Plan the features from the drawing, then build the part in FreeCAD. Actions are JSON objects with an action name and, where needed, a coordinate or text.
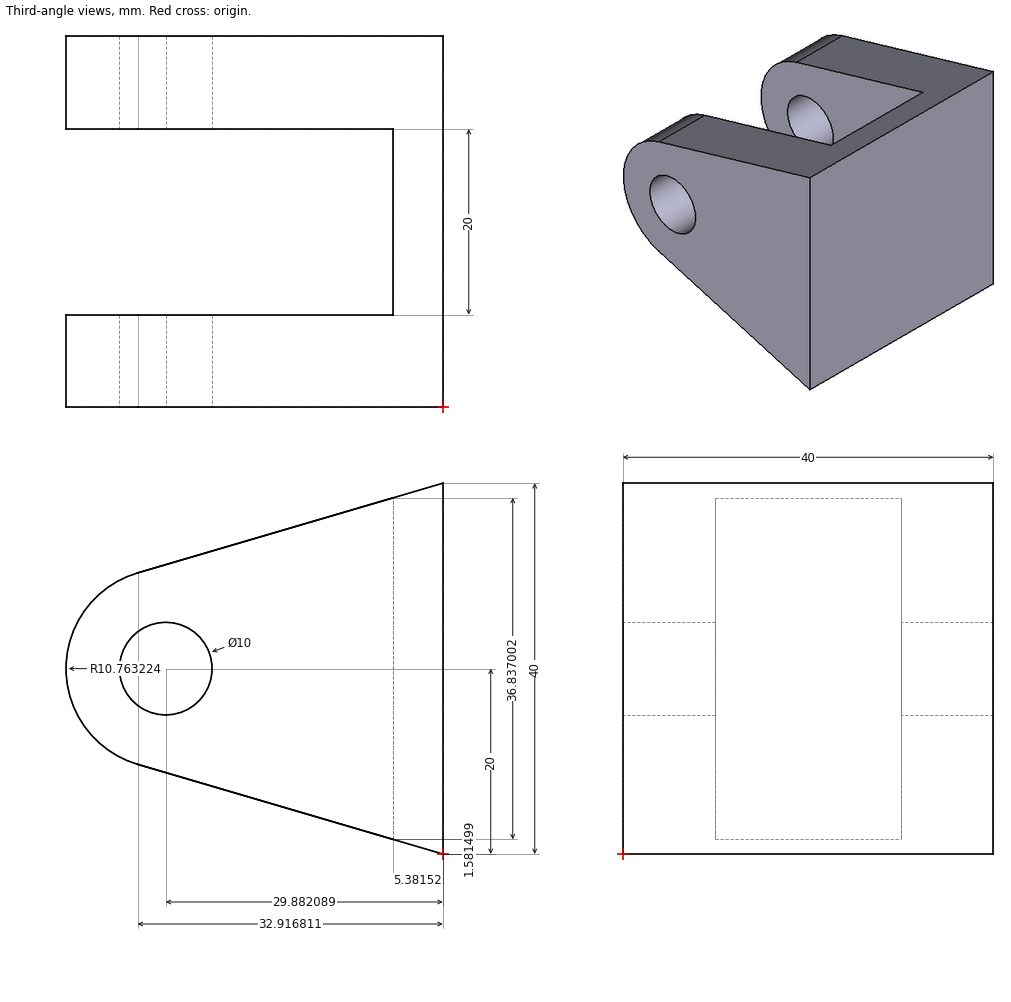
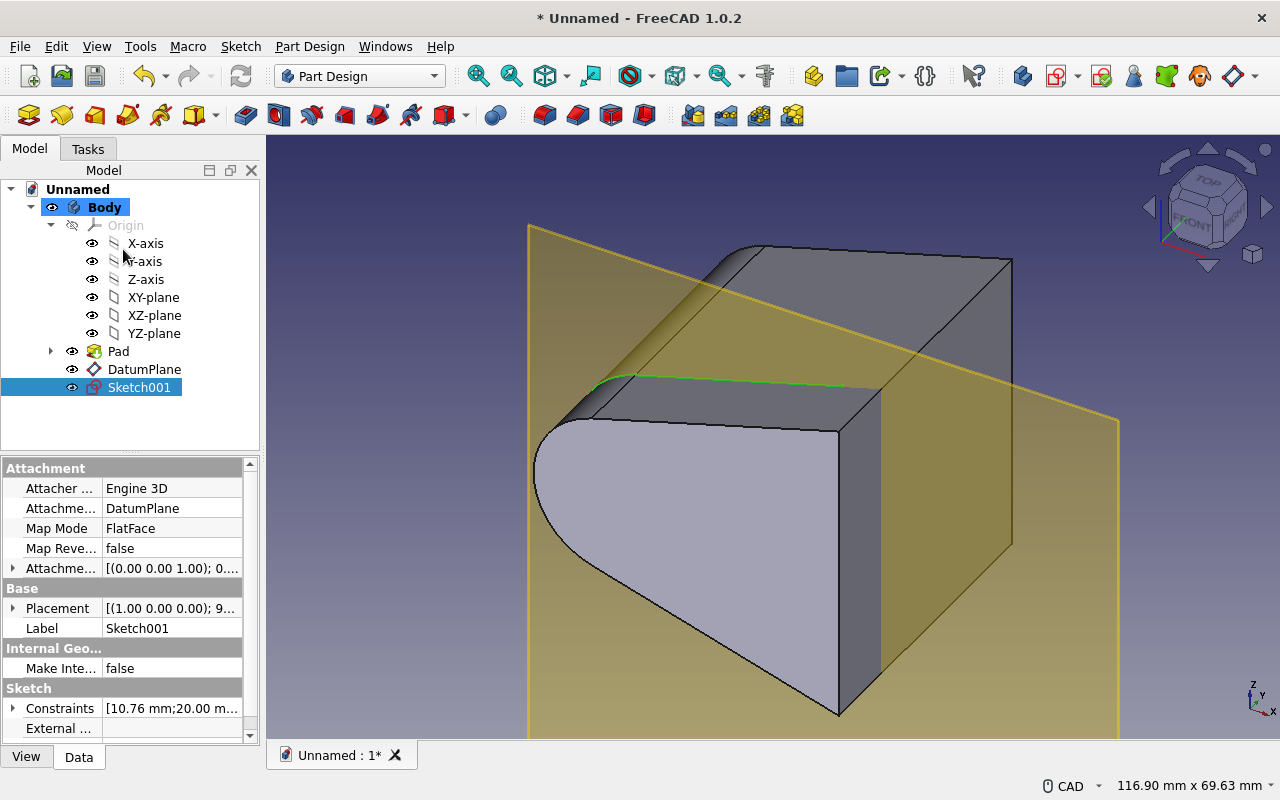
{"action": "left_click", "coordinate": [246, 116]}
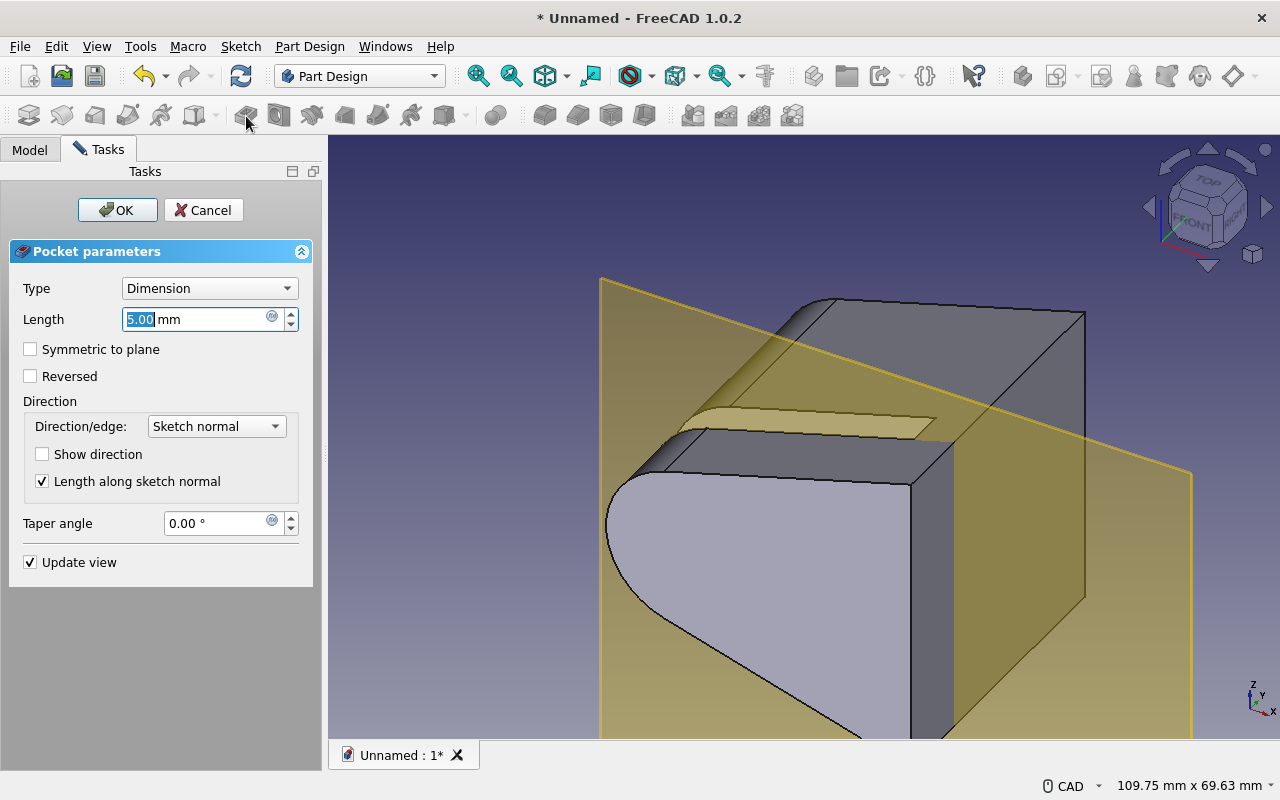
{"action": "type", "text": "20"}
{"action": "key", "text": "Tab"}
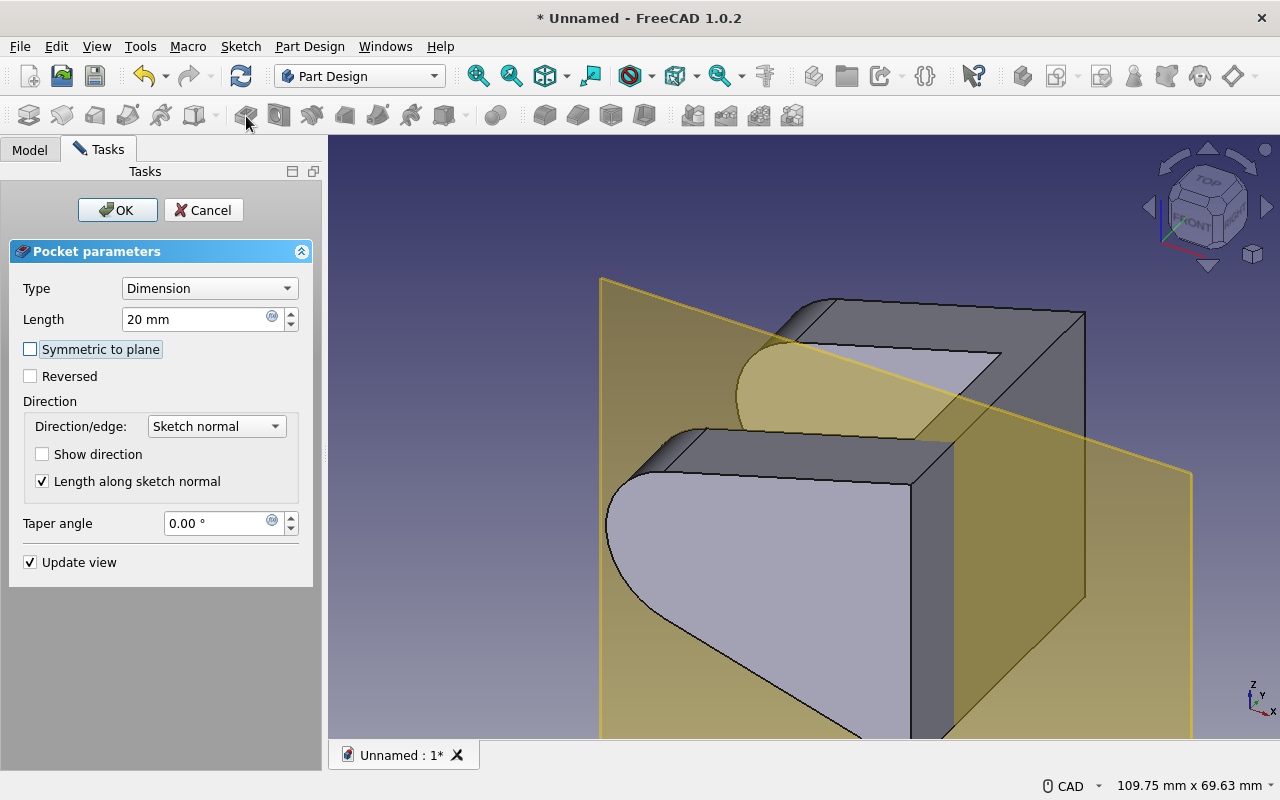
{"action": "left_click", "coordinate": [118, 210]}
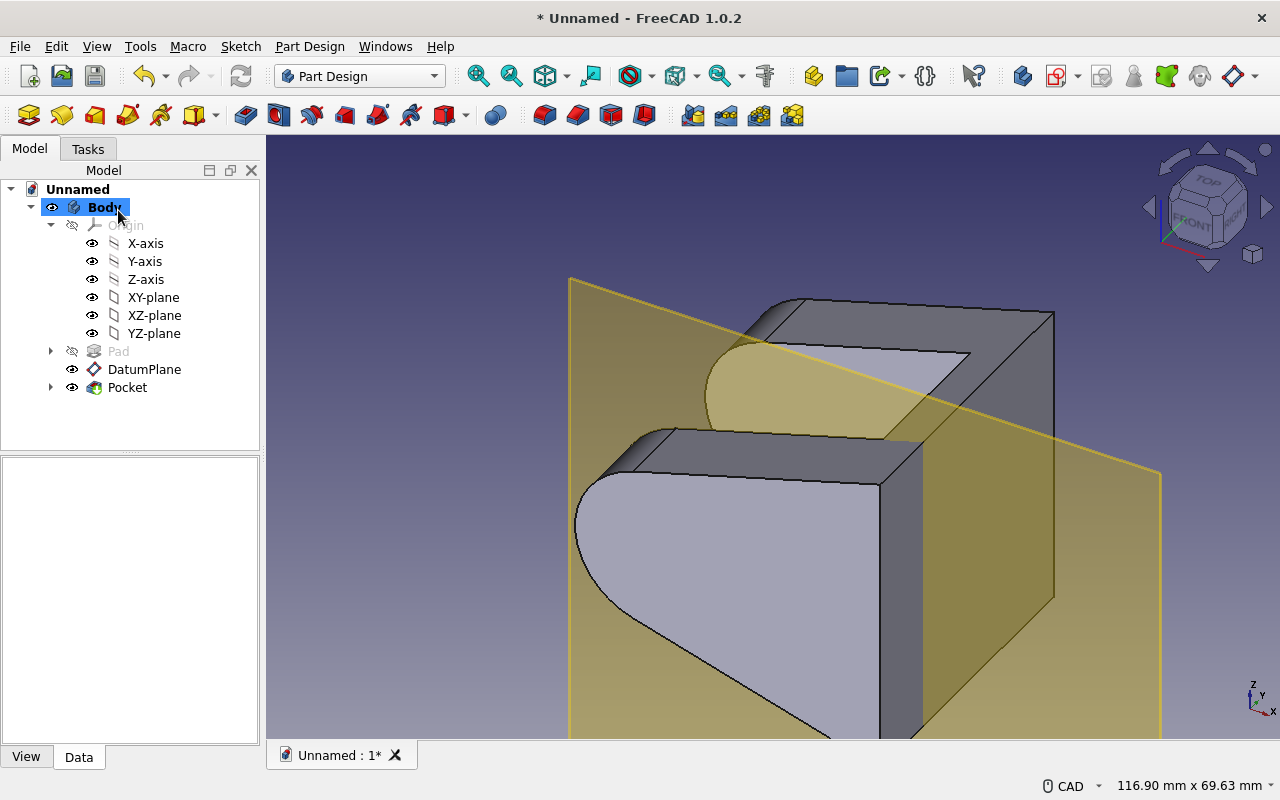
{"action": "left_click", "coordinate": [117, 369]}
{"action": "key", "text": "space"}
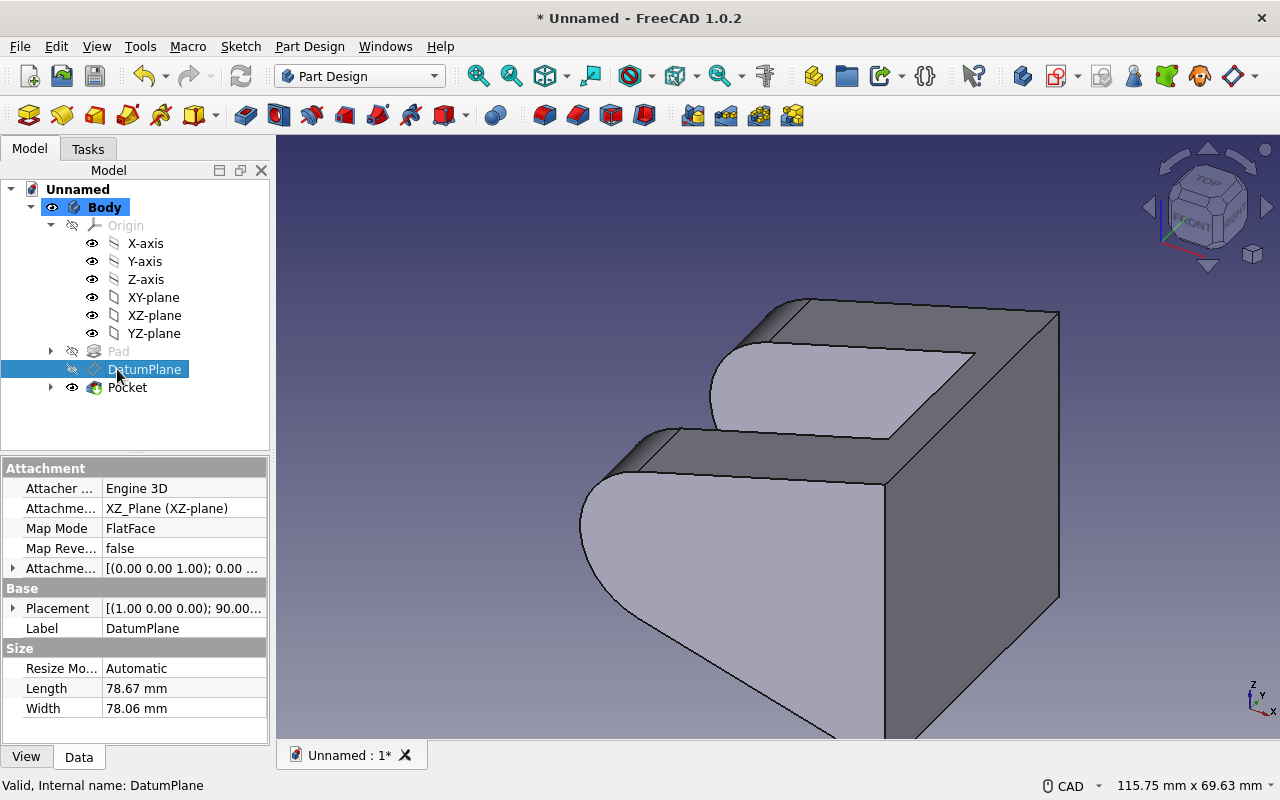
{"action": "left_click", "coordinate": [479, 76]}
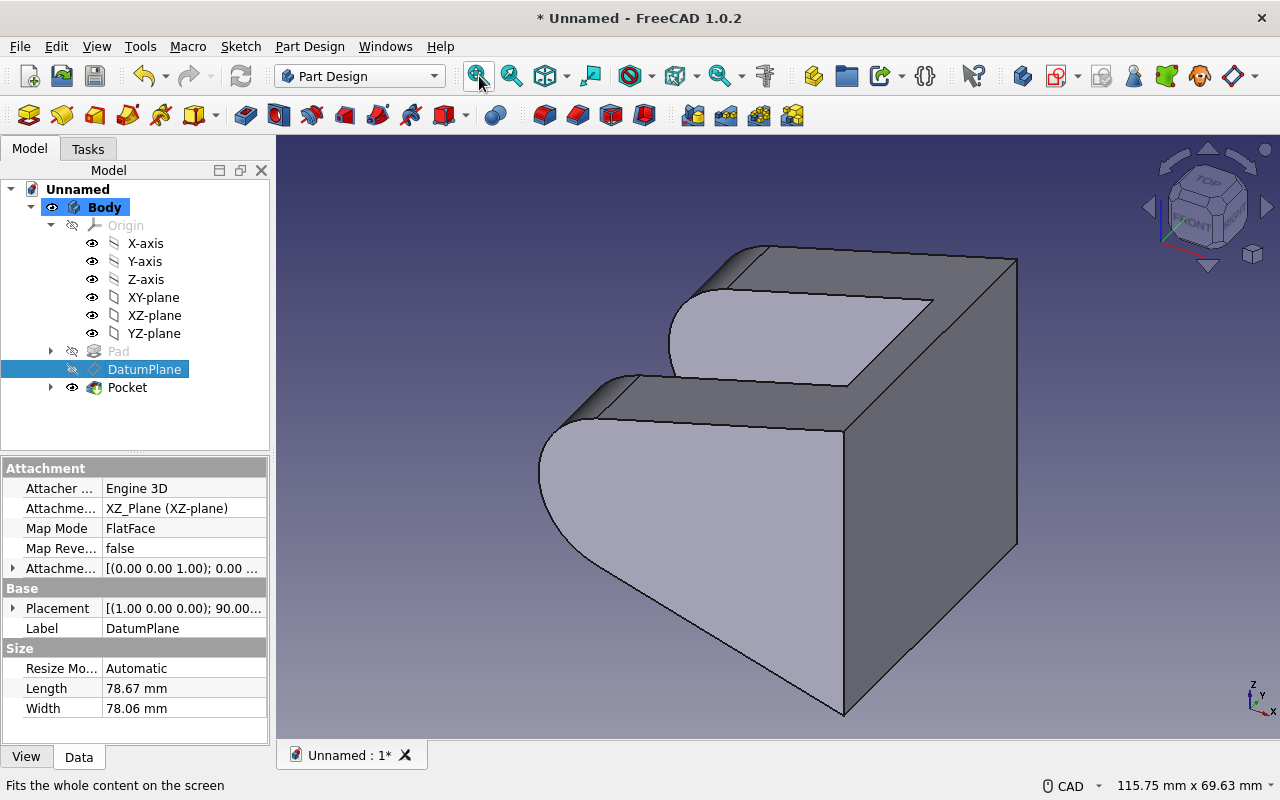
{"action": "left_click", "coordinate": [137, 315]}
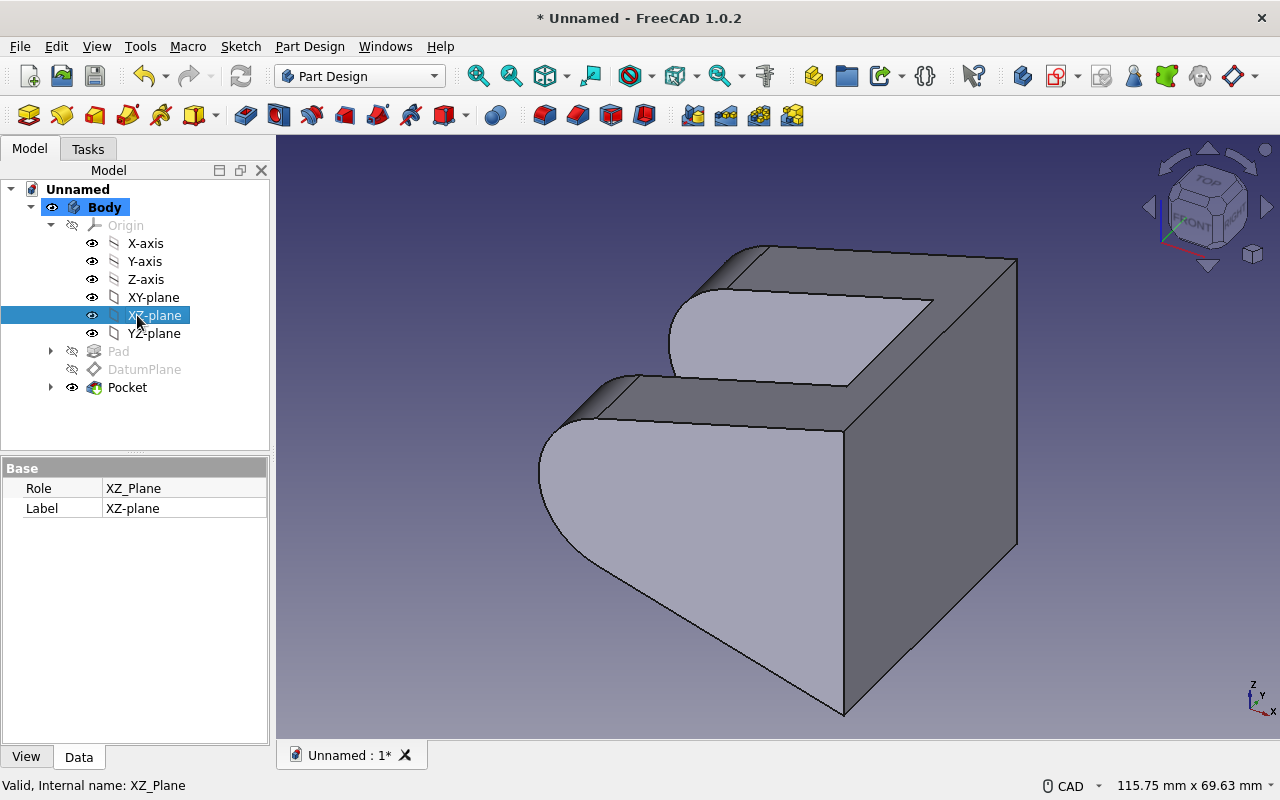
{"action": "left_click", "coordinate": [1232, 76]}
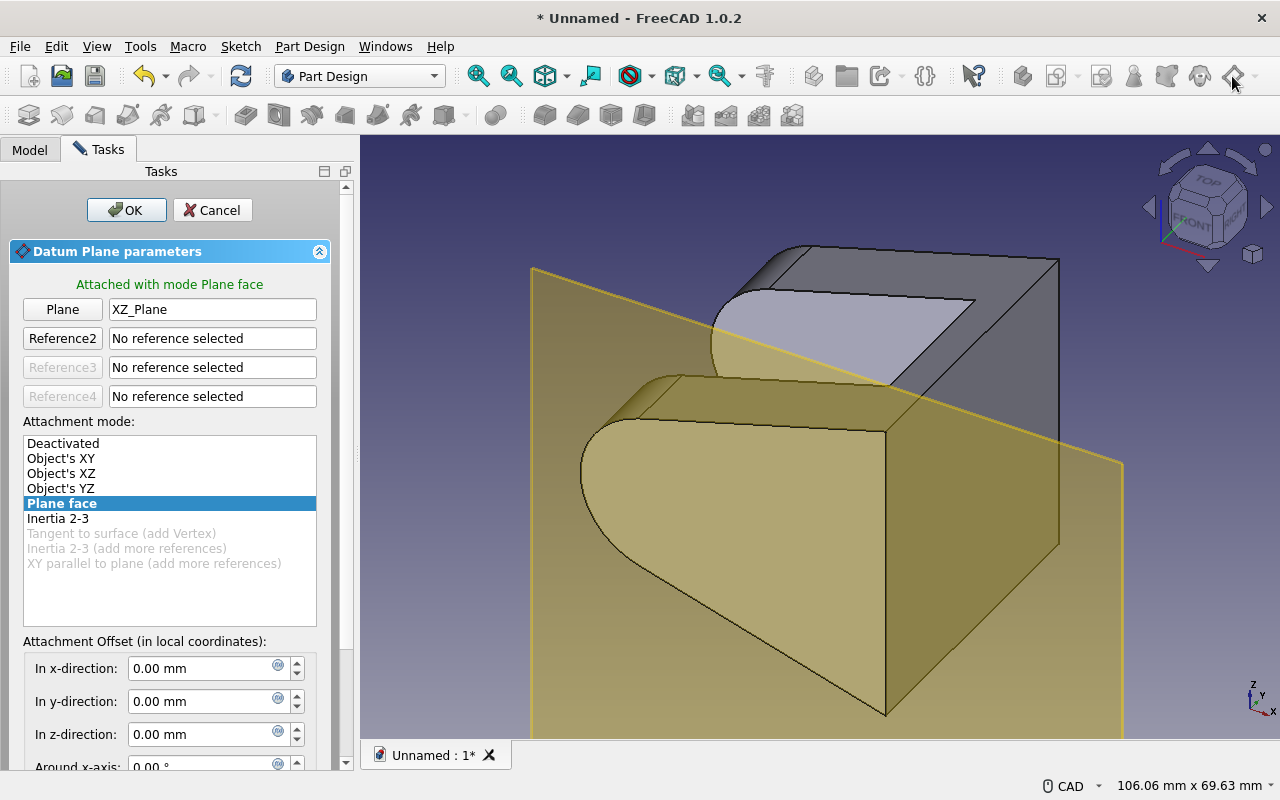
{"action": "triple_click", "coordinate": [210, 734]}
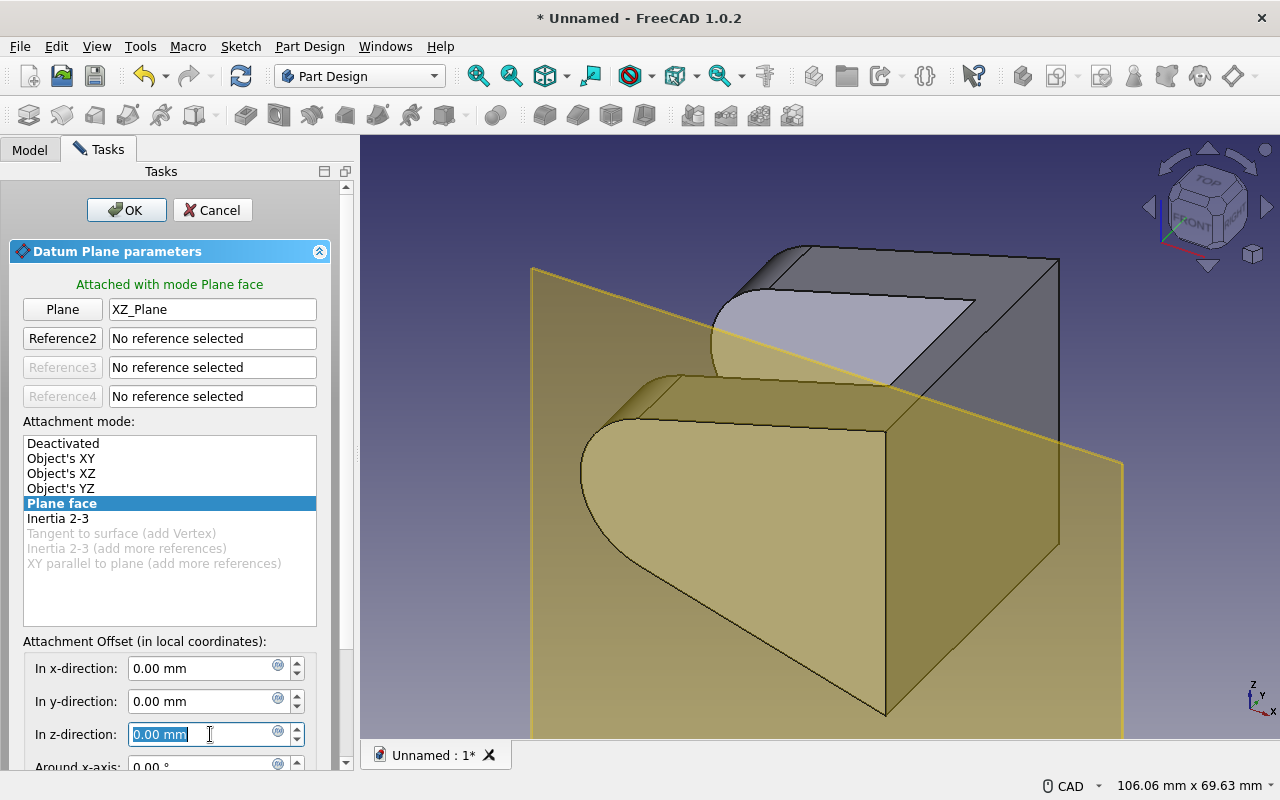
{"action": "type", "text": "-10"}
{"action": "key", "text": "Tab"}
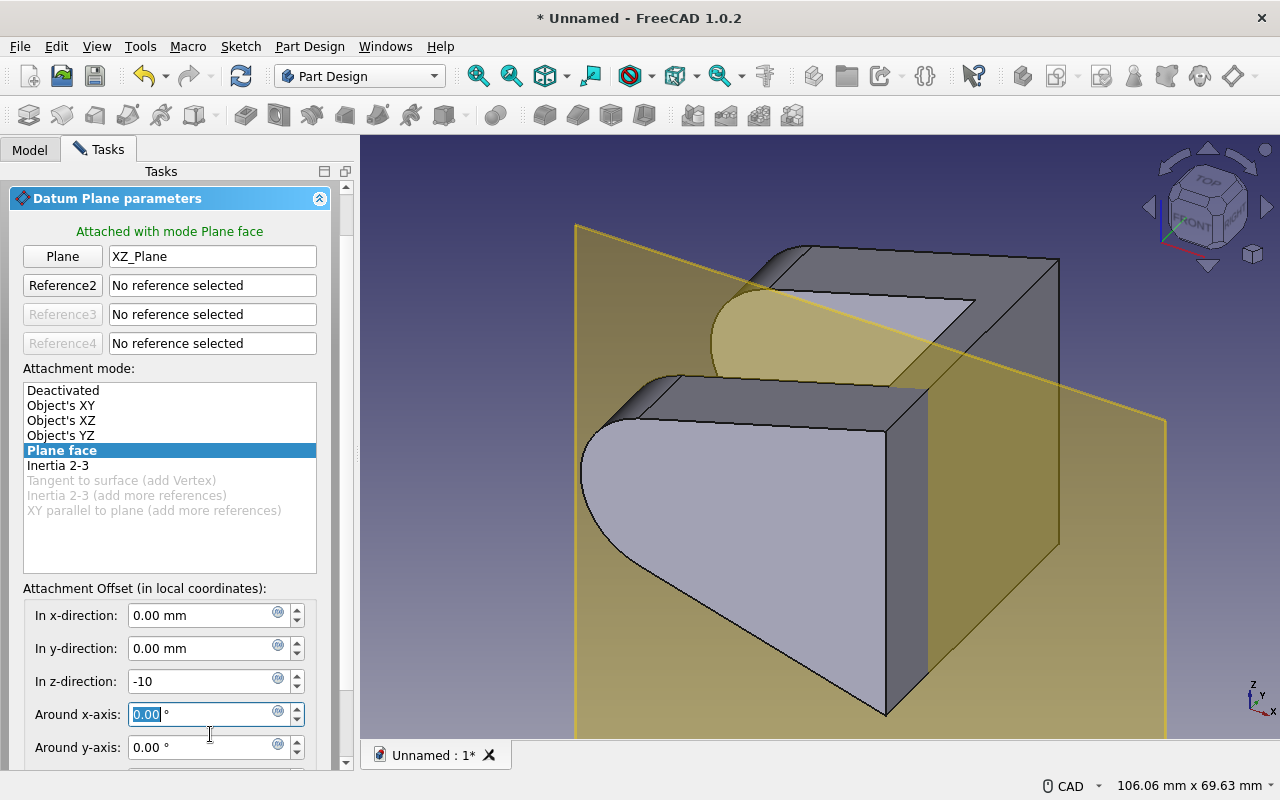
{"action": "scroll", "coordinate": [346, 476], "scroll_direction": "up", "scroll_amount": 2}